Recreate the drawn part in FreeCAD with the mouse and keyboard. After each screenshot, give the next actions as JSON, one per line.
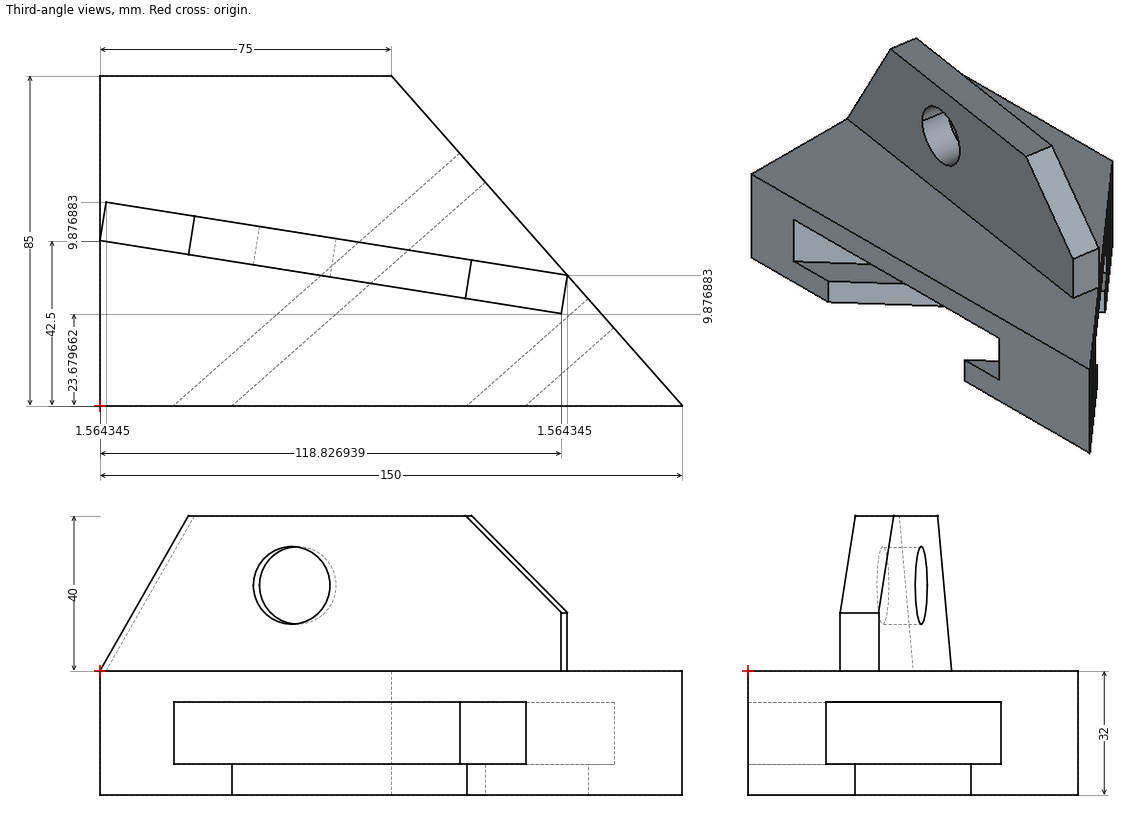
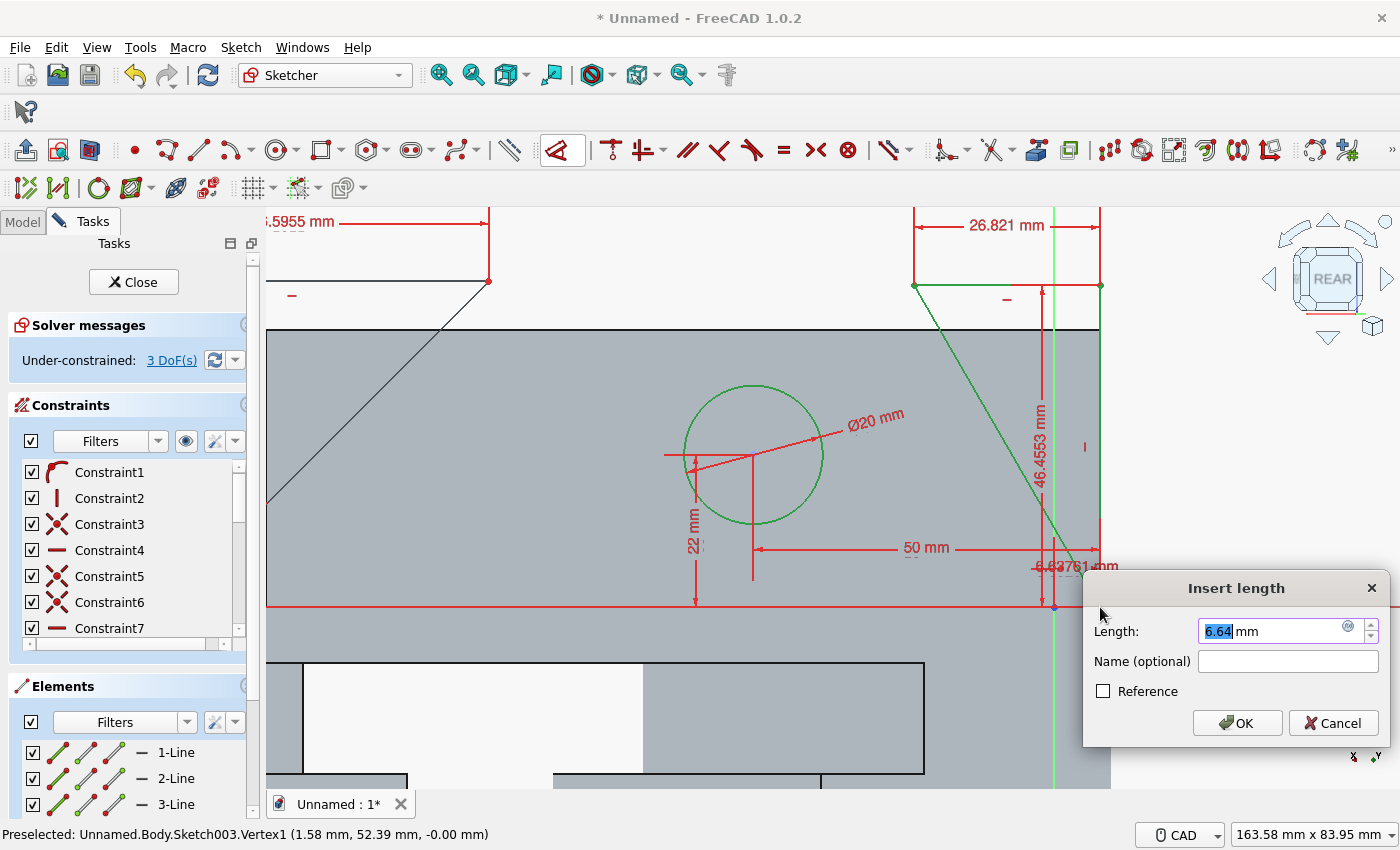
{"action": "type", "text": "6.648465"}
{"action": "key", "text": "Return"}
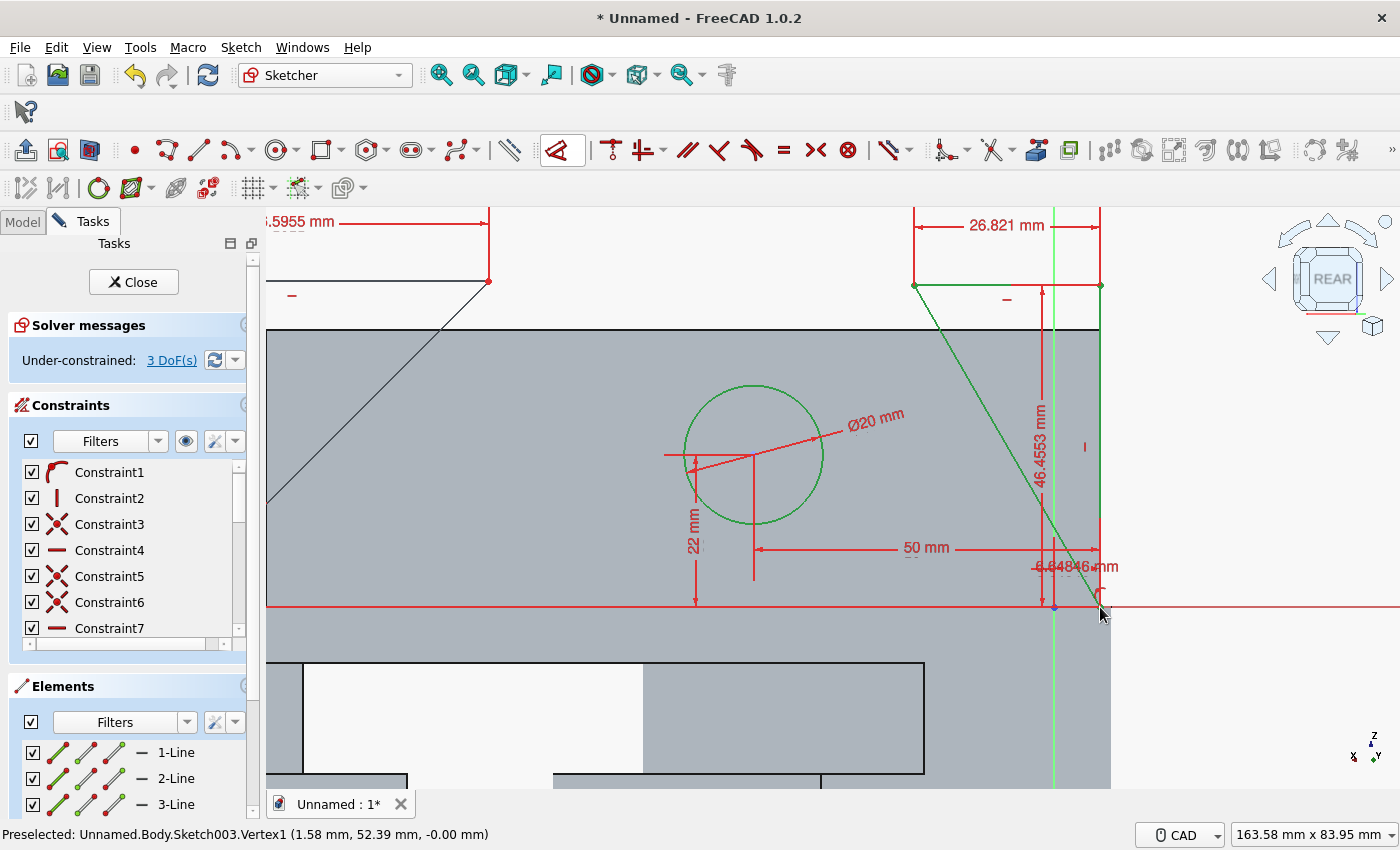
{"action": "left_click", "coordinate": [489, 281]}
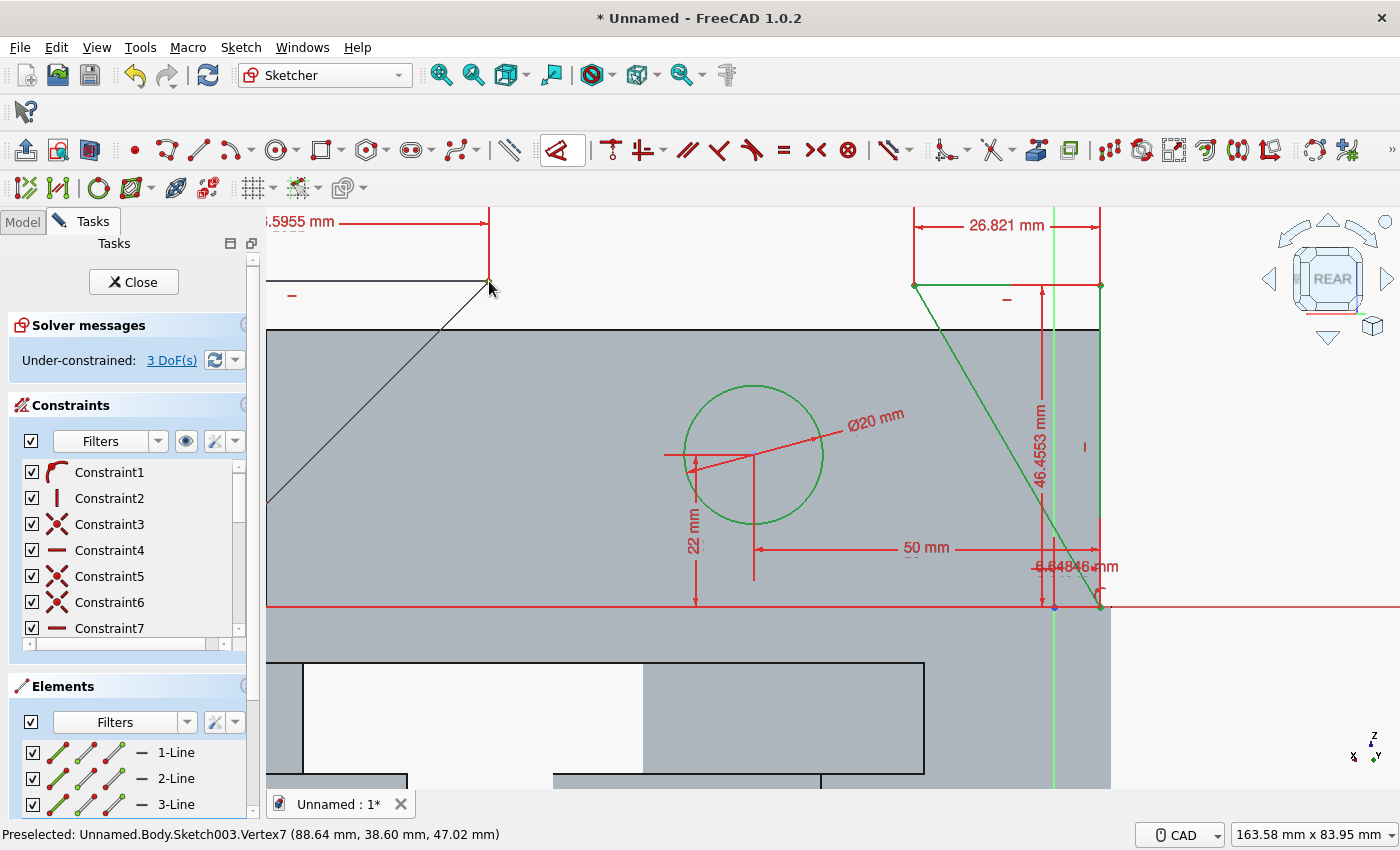
{"action": "left_click", "coordinate": [580, 150]}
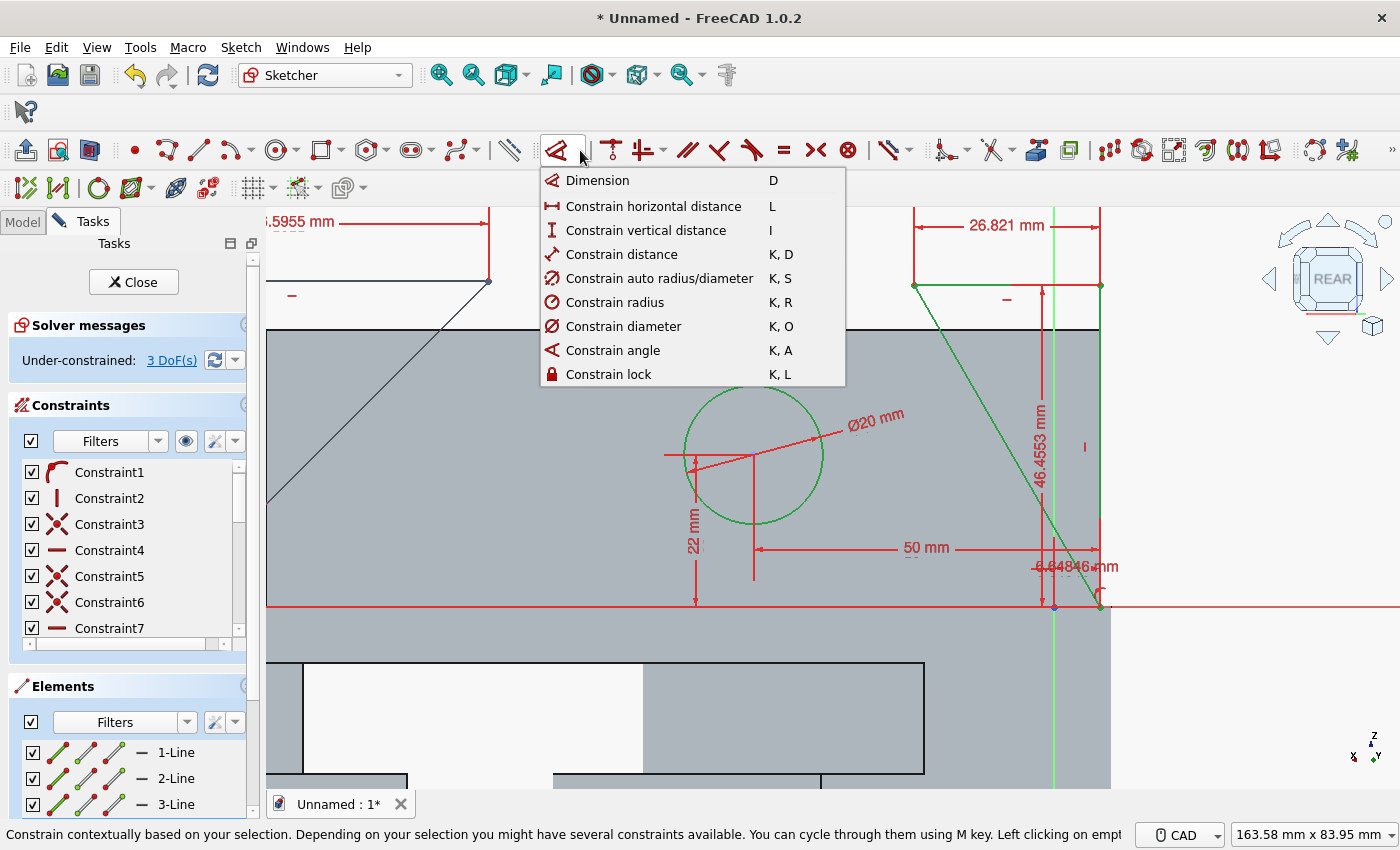
{"action": "left_click", "coordinate": [693, 206]}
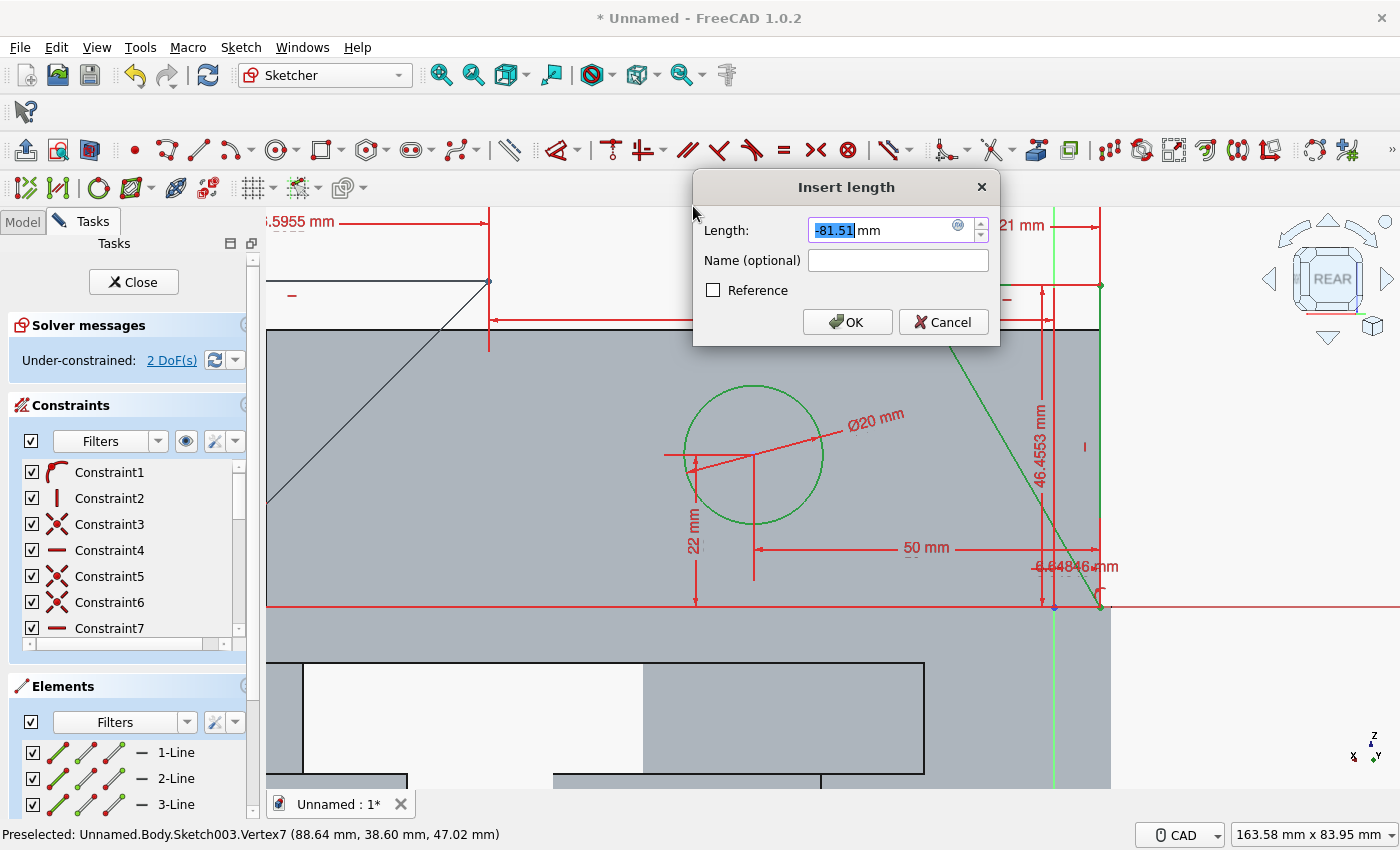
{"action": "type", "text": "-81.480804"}
{"action": "key", "text": "Return"}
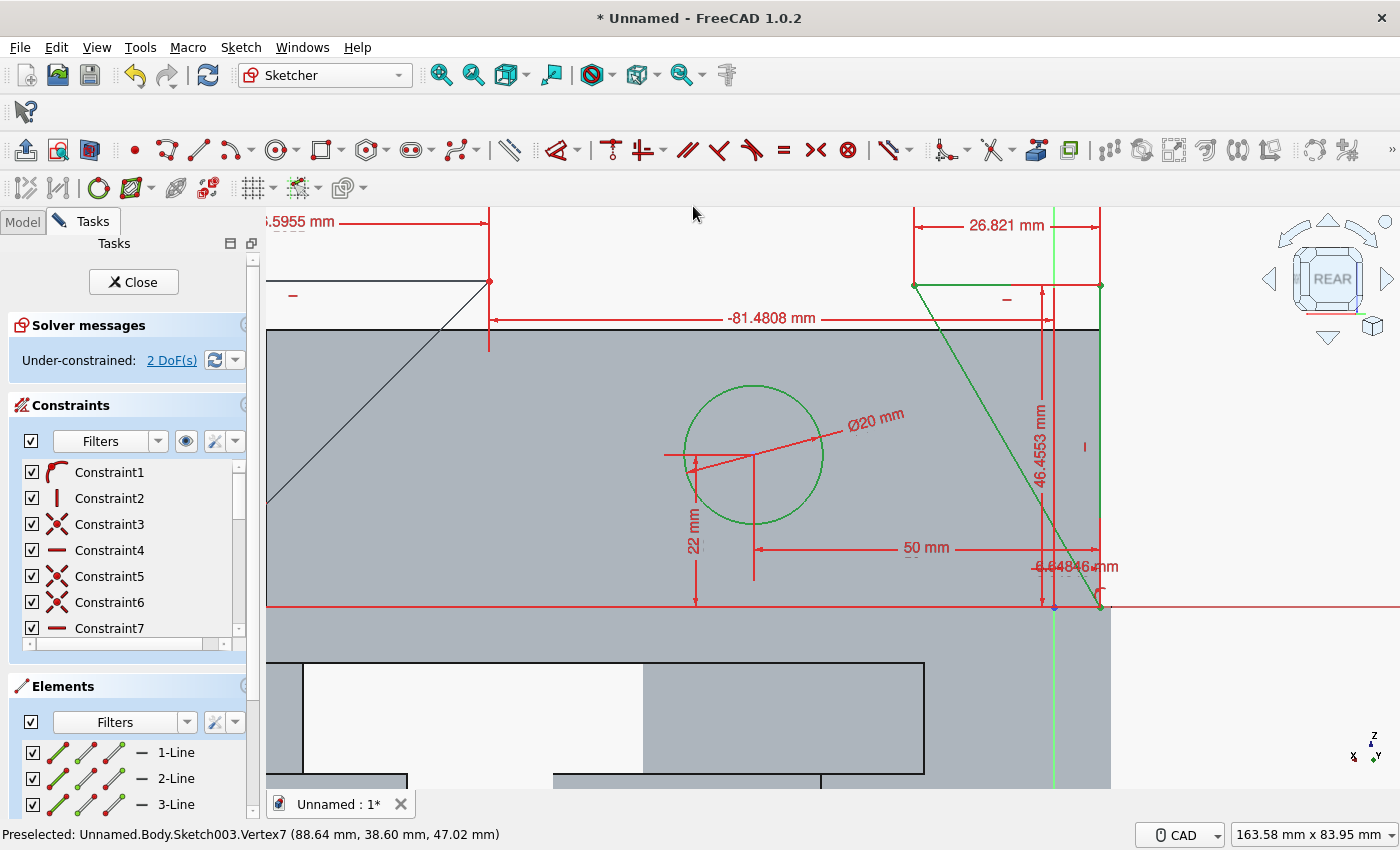
{"action": "left_click", "coordinate": [489, 281]}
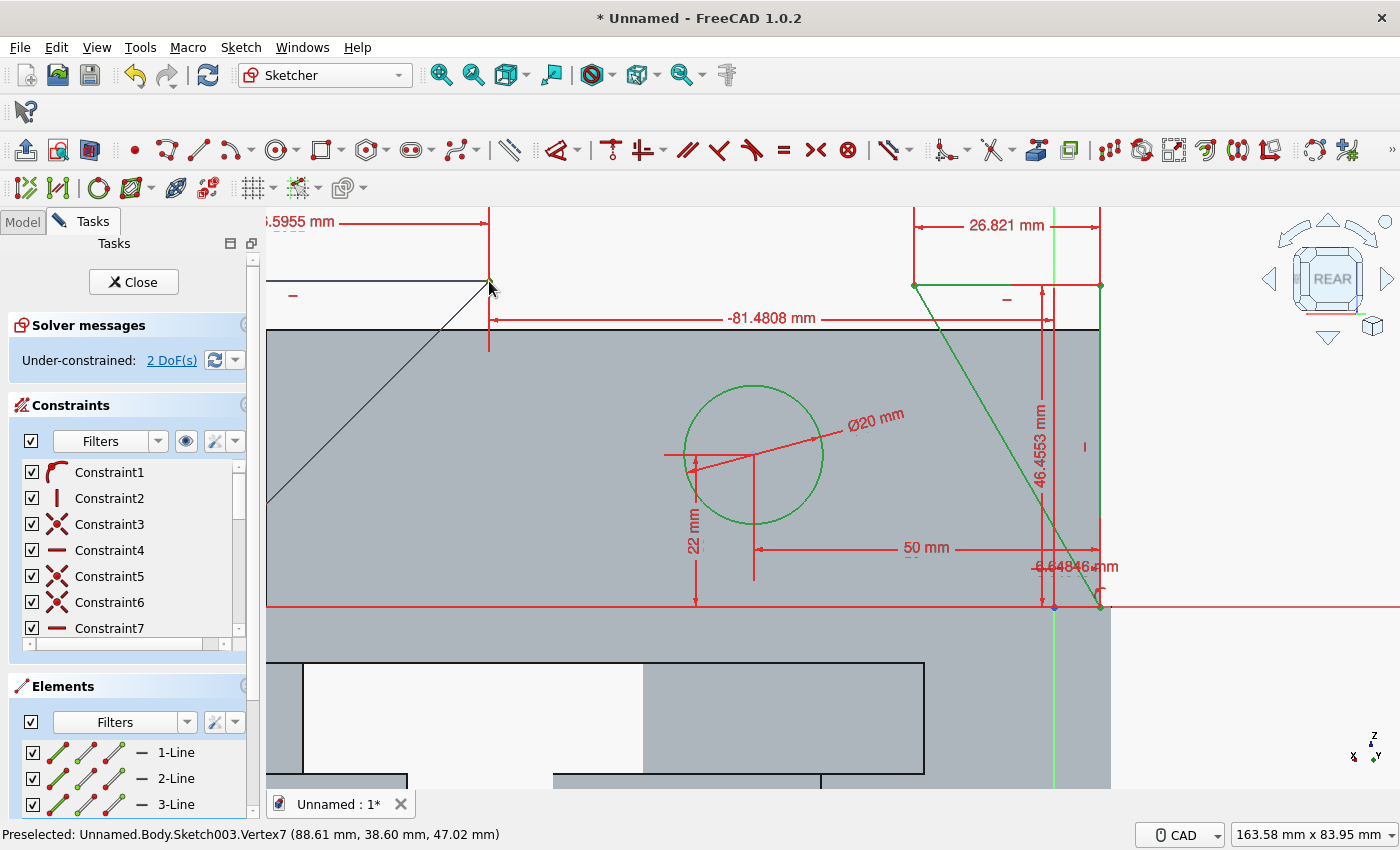
{"action": "left_click", "coordinate": [580, 150]}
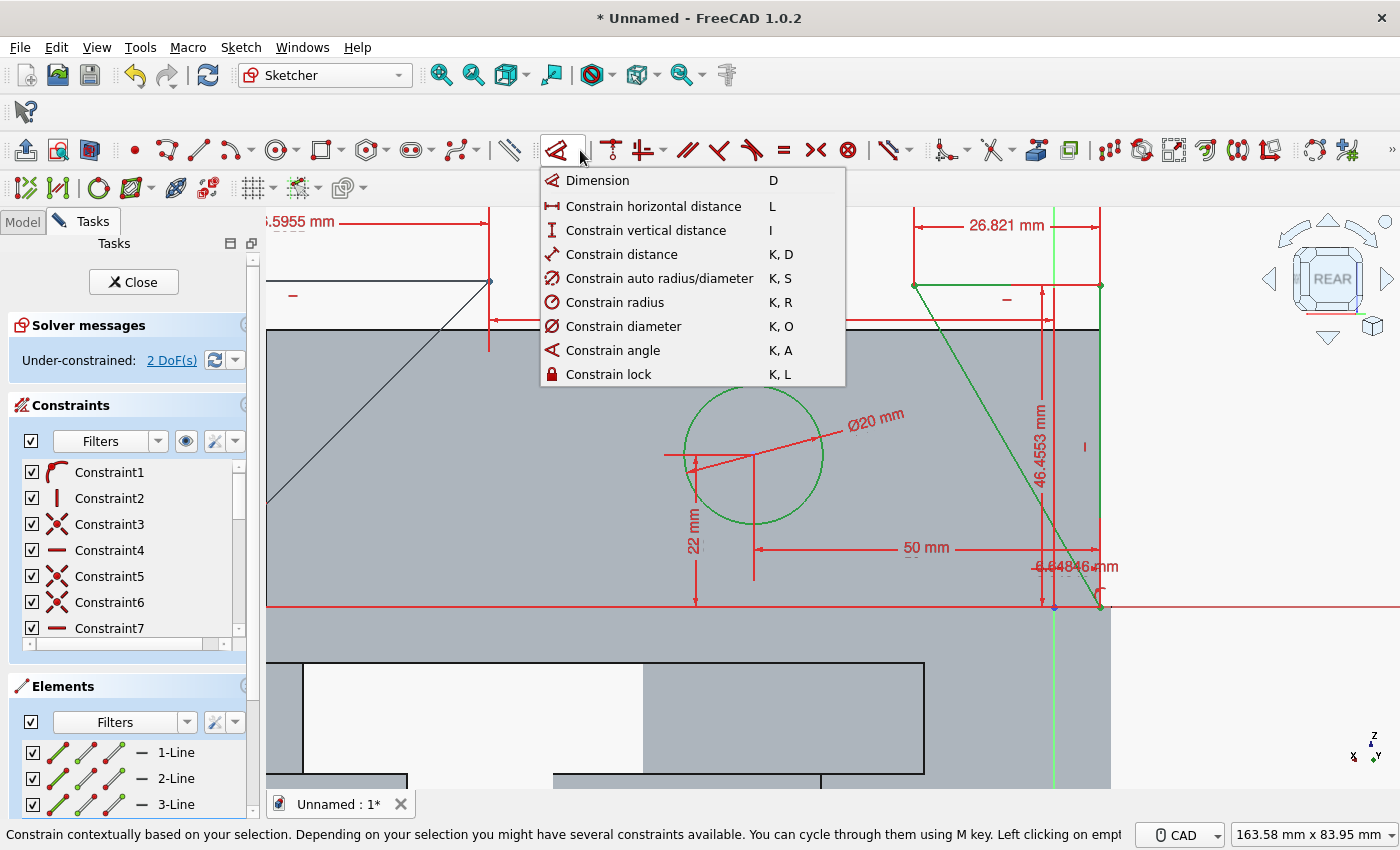
{"action": "left_click", "coordinate": [693, 230]}